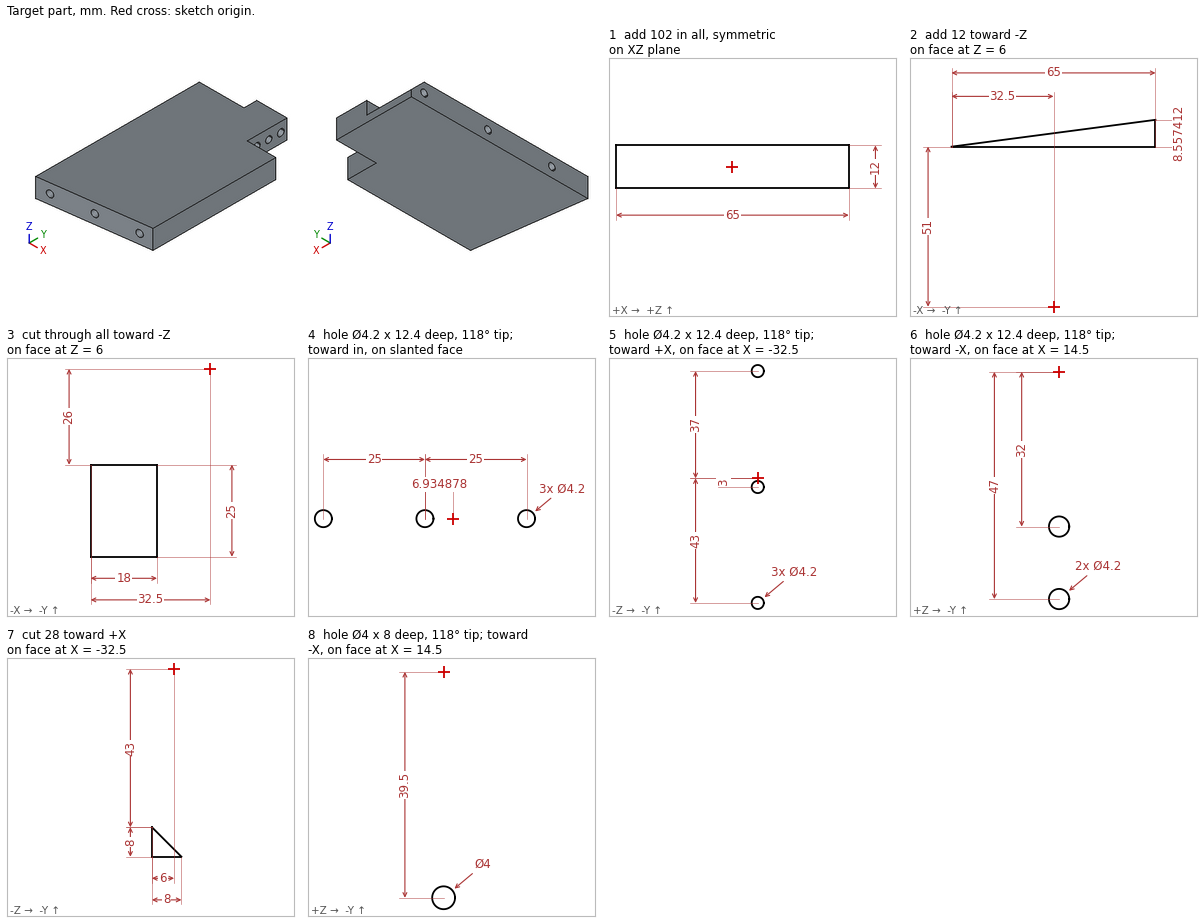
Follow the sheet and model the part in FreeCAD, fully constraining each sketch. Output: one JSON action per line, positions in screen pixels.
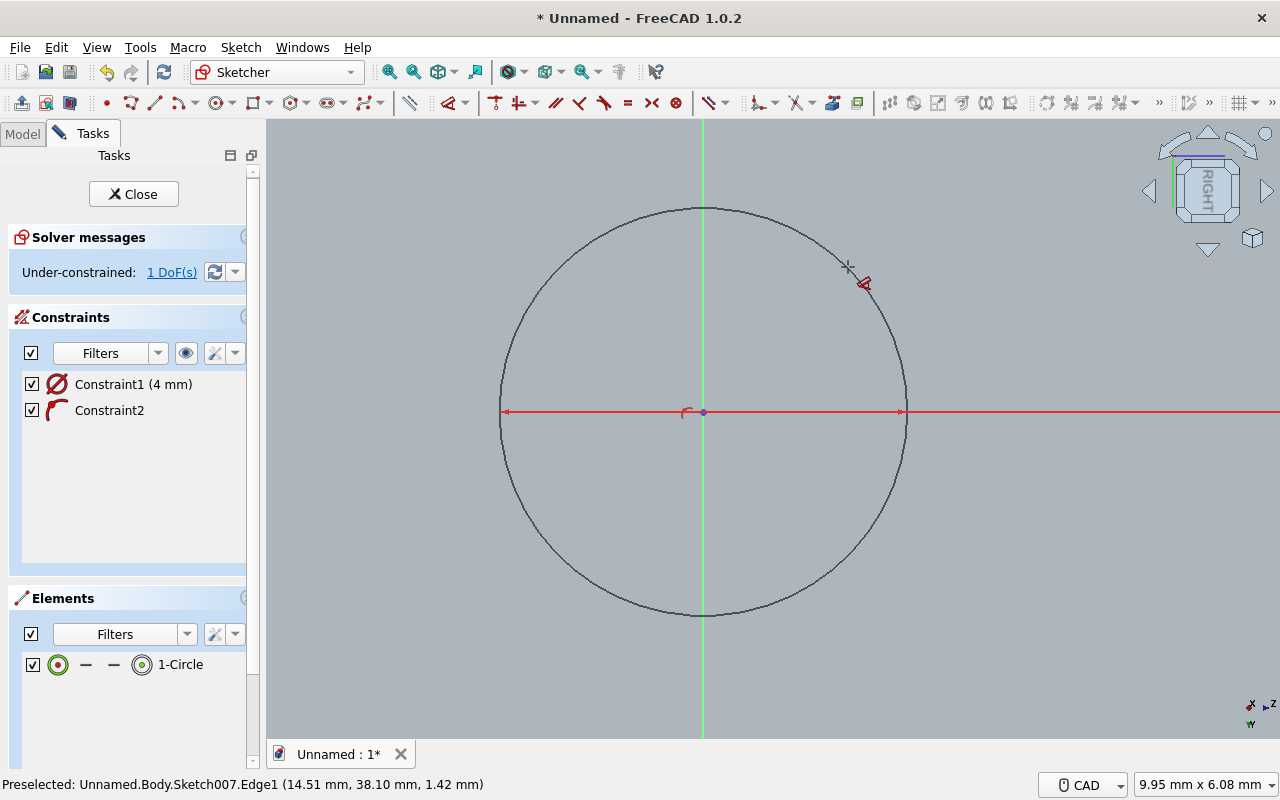
{"action": "left_click", "coordinate": [703, 412]}
{"action": "left_click", "coordinate": [737, 280]}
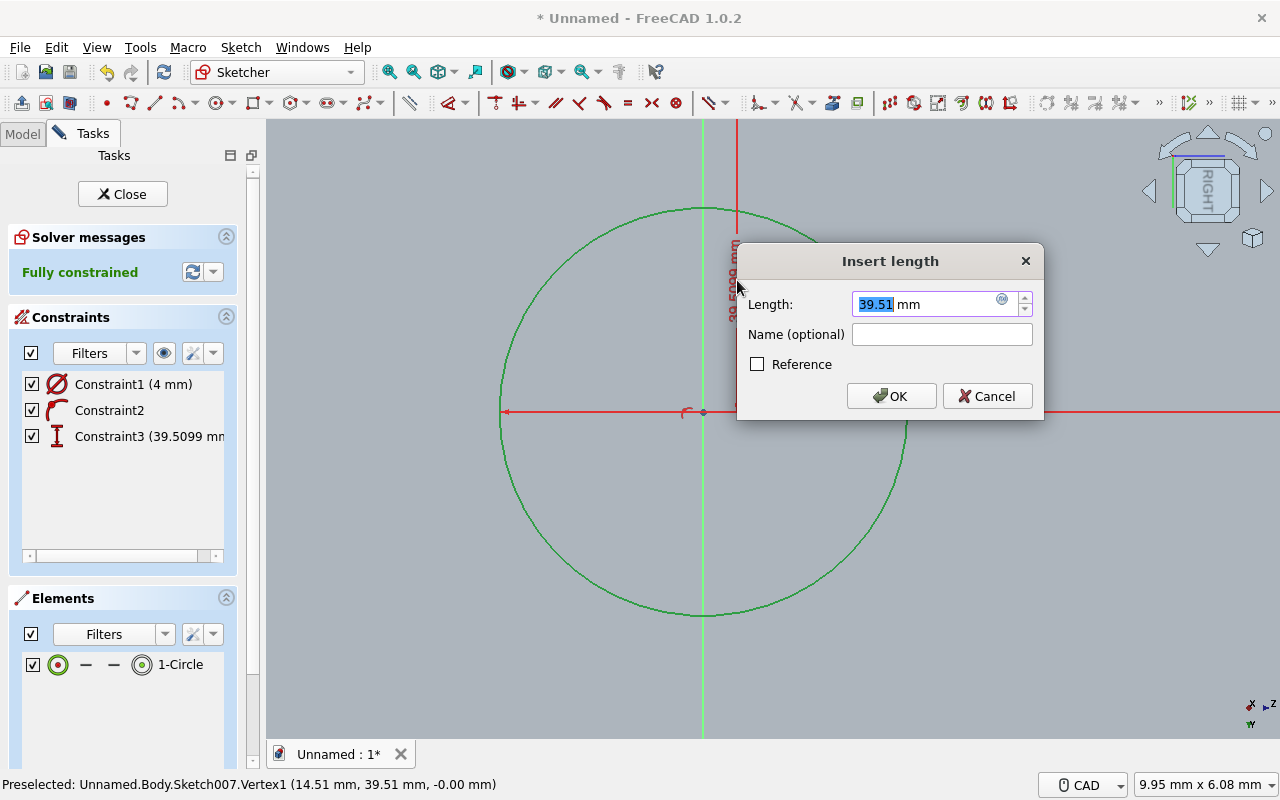
{"action": "type", "text": "39.5"}
{"action": "key", "text": "Return"}
{"action": "key", "text": "Escape"}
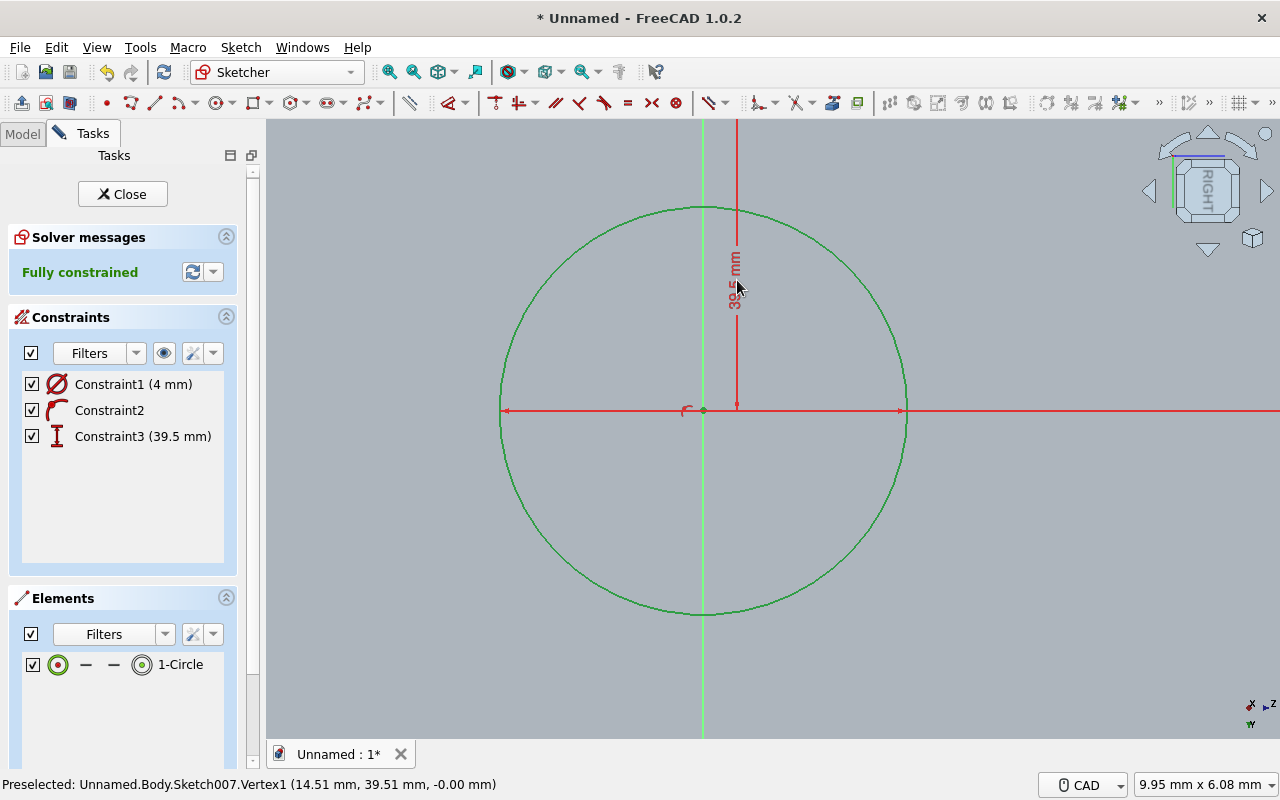
{"action": "left_click", "coordinate": [123, 194]}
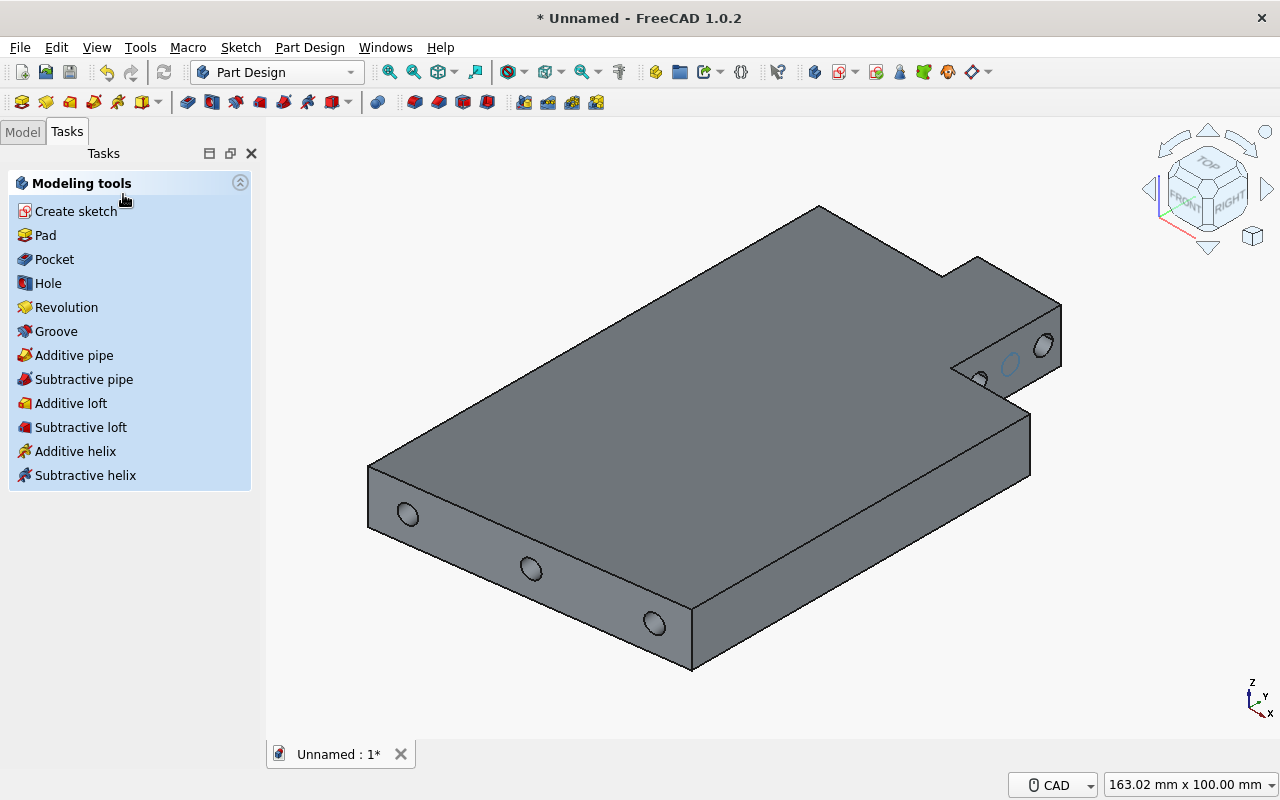
{"action": "left_click", "coordinate": [212, 102]}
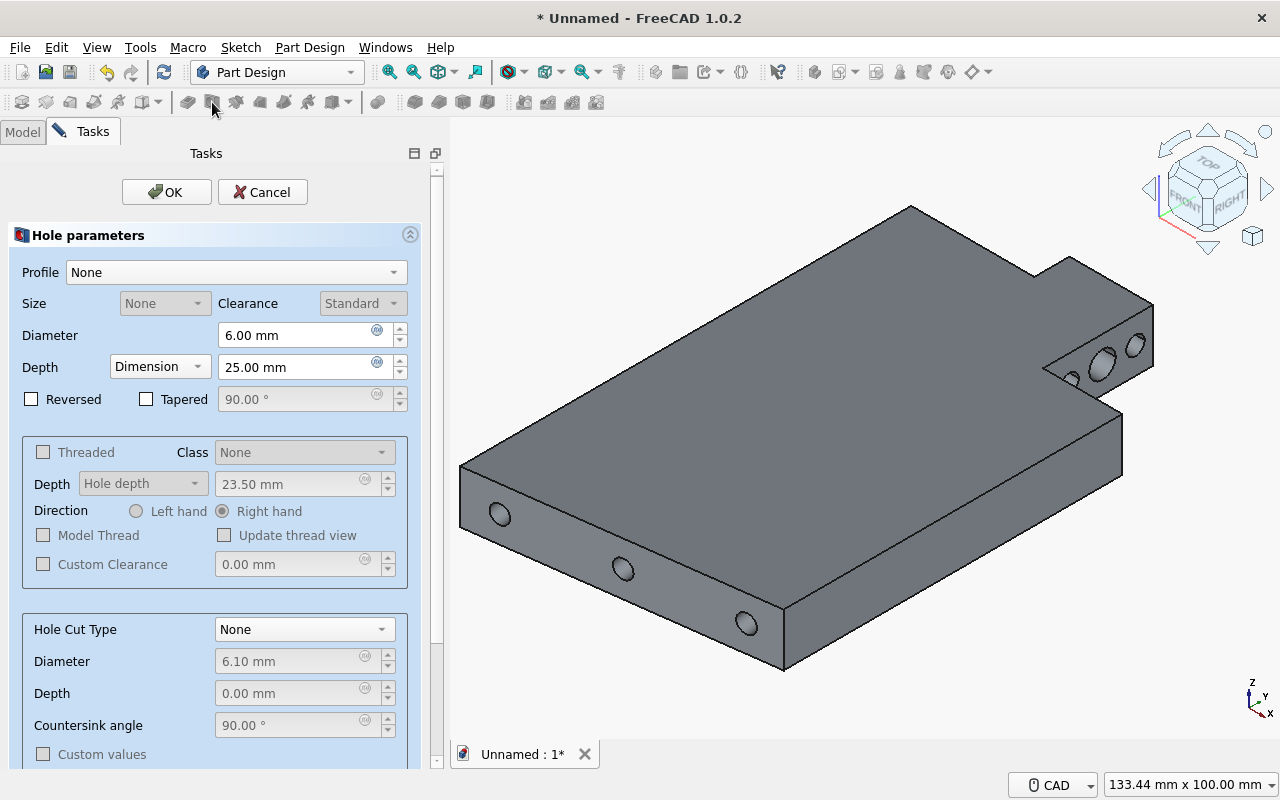
{"action": "triple_click", "coordinate": [305, 335]}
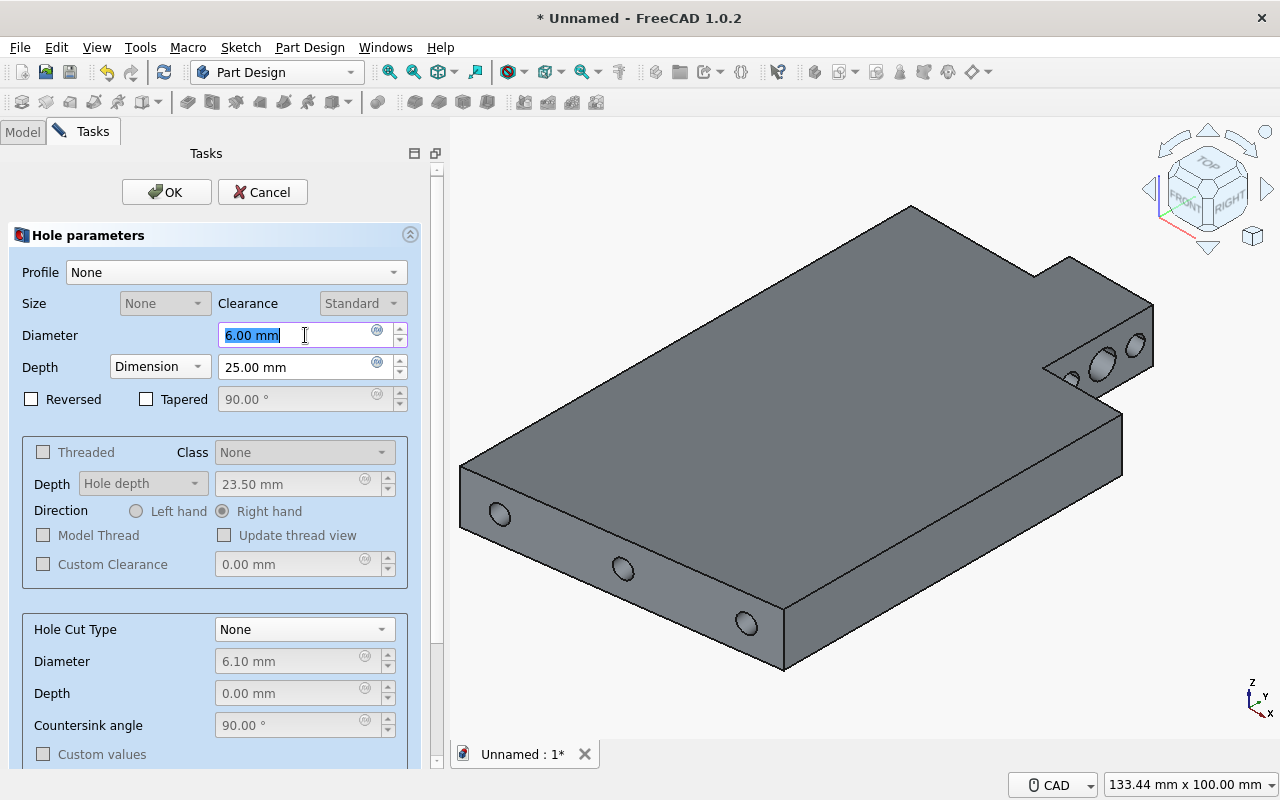
{"action": "type", "text": "4"}
{"action": "key", "text": "Tab"}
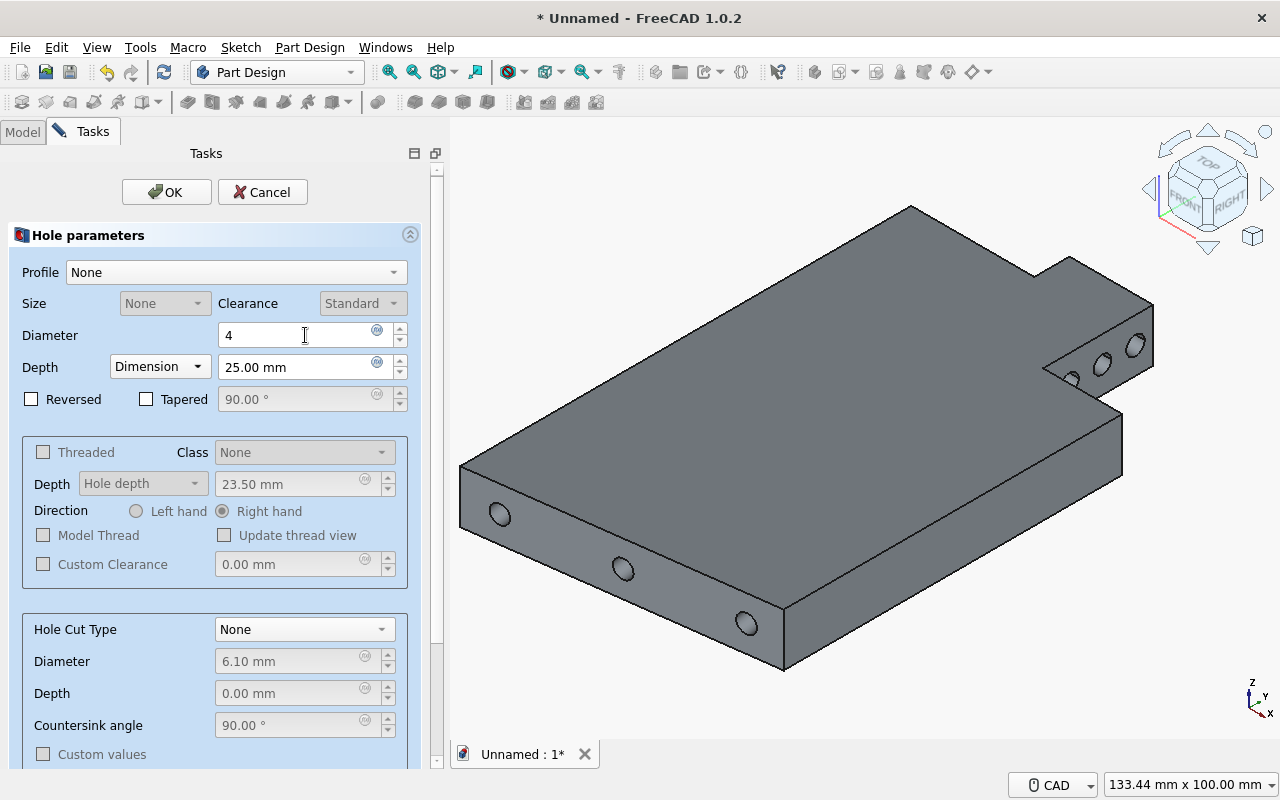
{"action": "triple_click", "coordinate": [305, 367]}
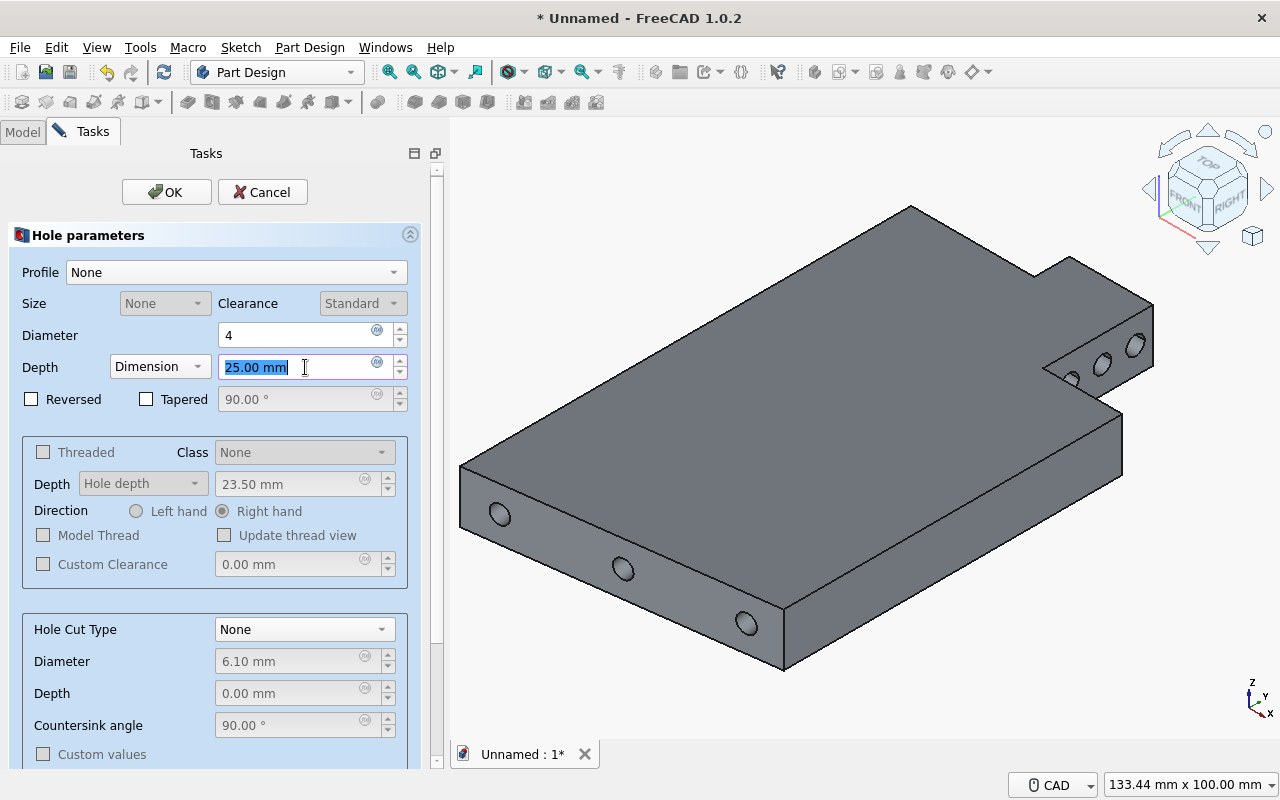
{"action": "type", "text": "8"}
{"action": "key", "text": "Tab"}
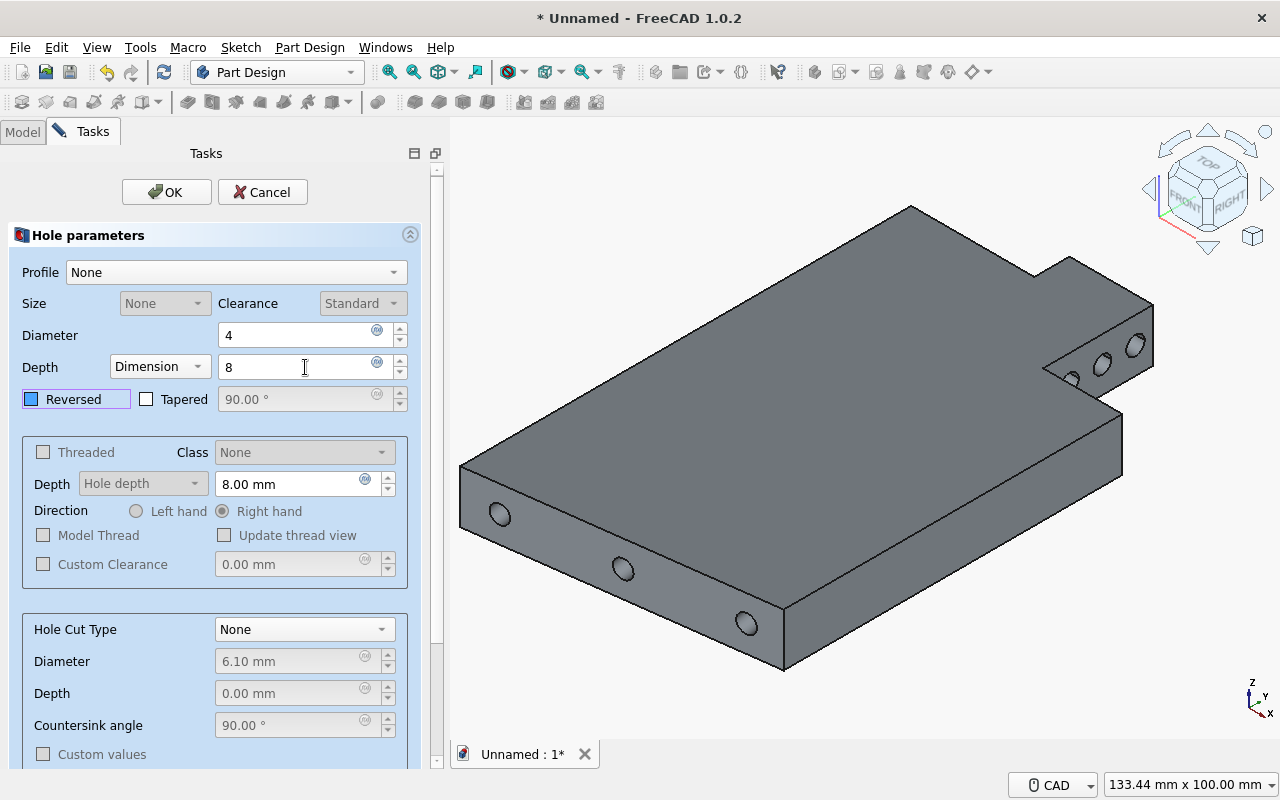
{"action": "left_click", "coordinate": [167, 192]}